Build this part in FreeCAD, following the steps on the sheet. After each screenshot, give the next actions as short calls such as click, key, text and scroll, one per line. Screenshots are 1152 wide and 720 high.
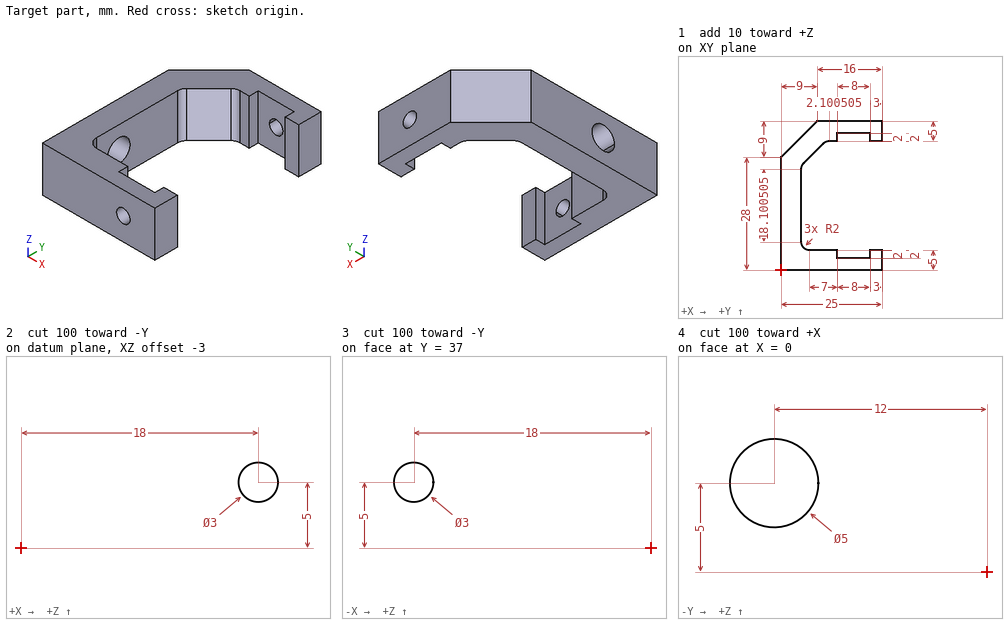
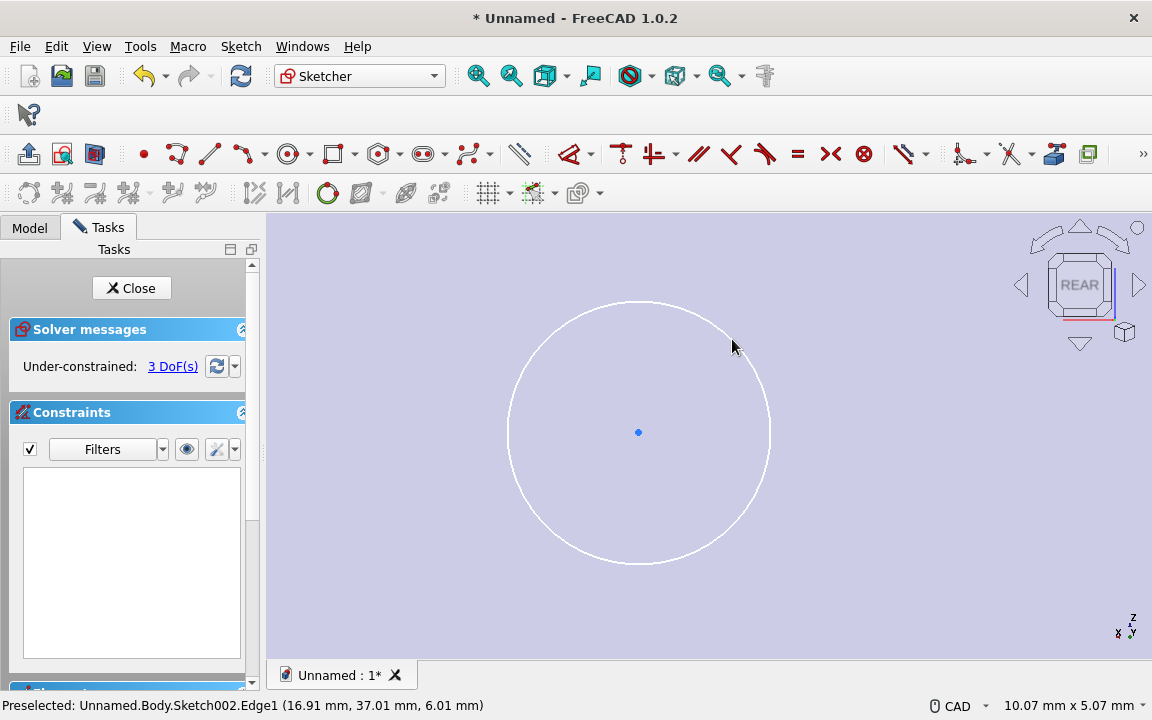
click(568, 154)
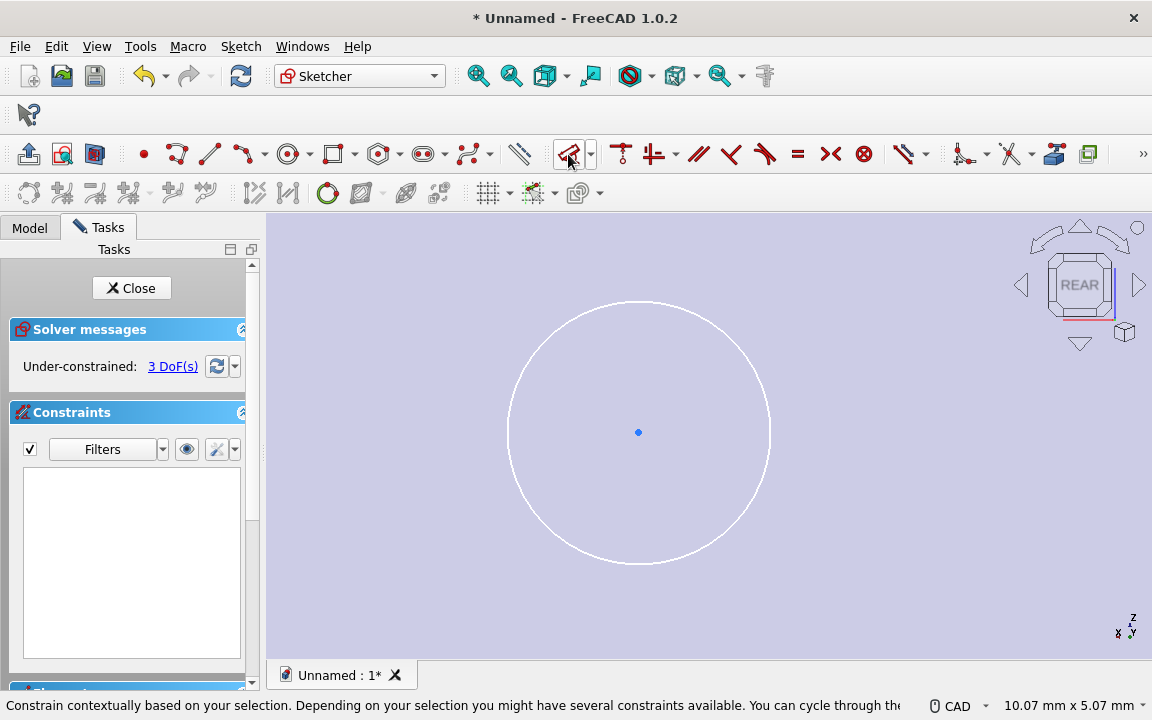
click(732, 340)
click(755, 317)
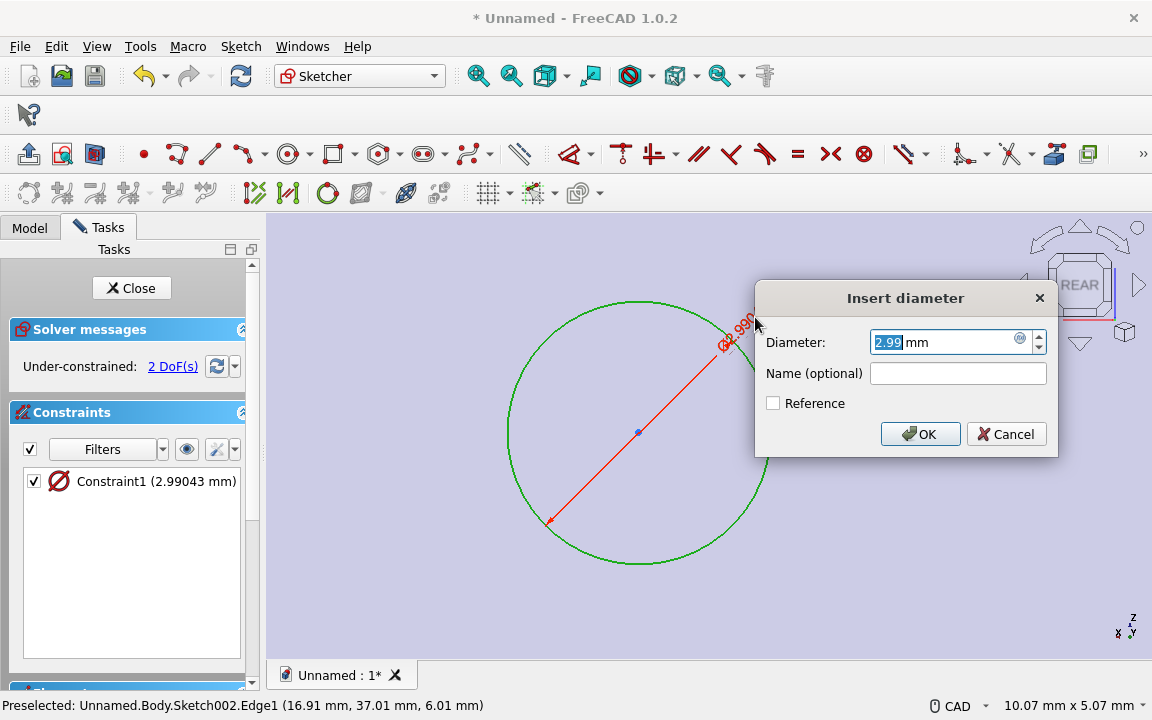
text(3)
key(Return)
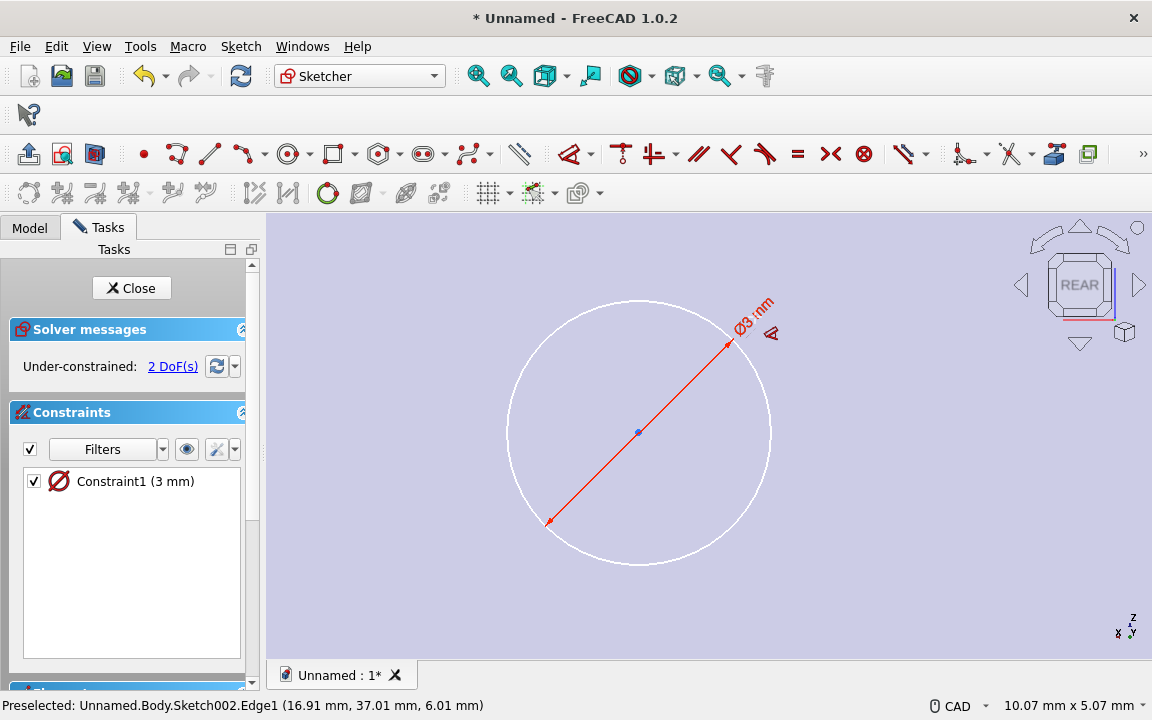
click(639, 433)
click(605, 532)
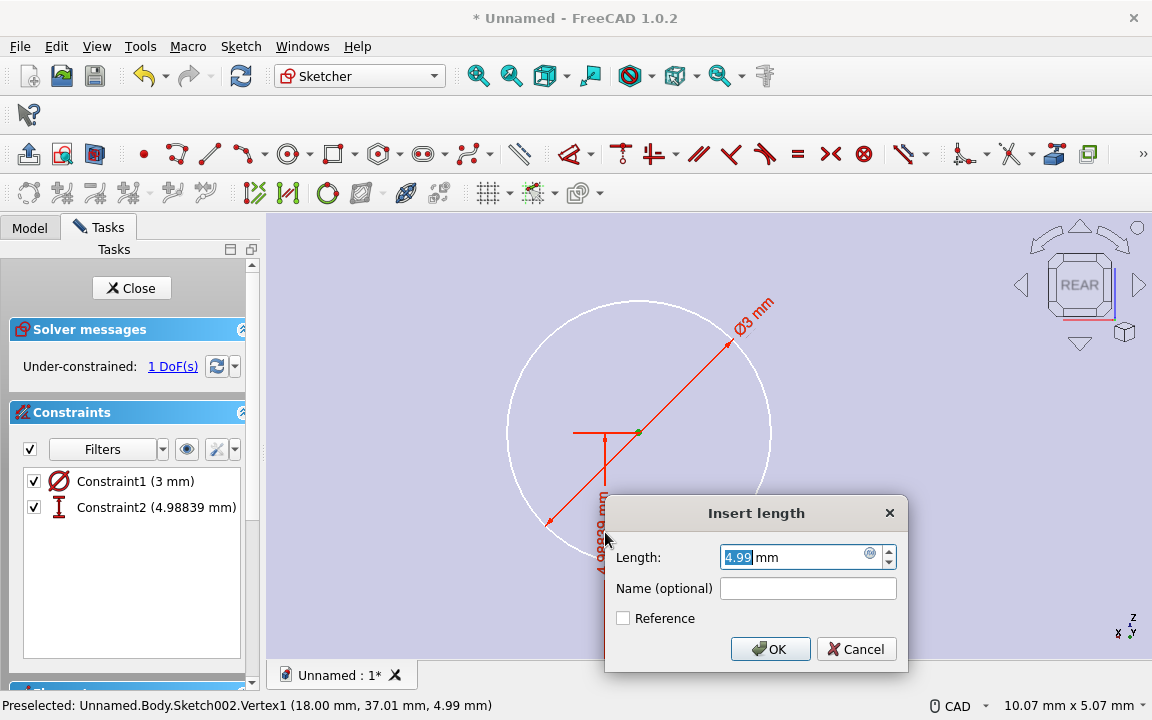
text(5)
key(Return)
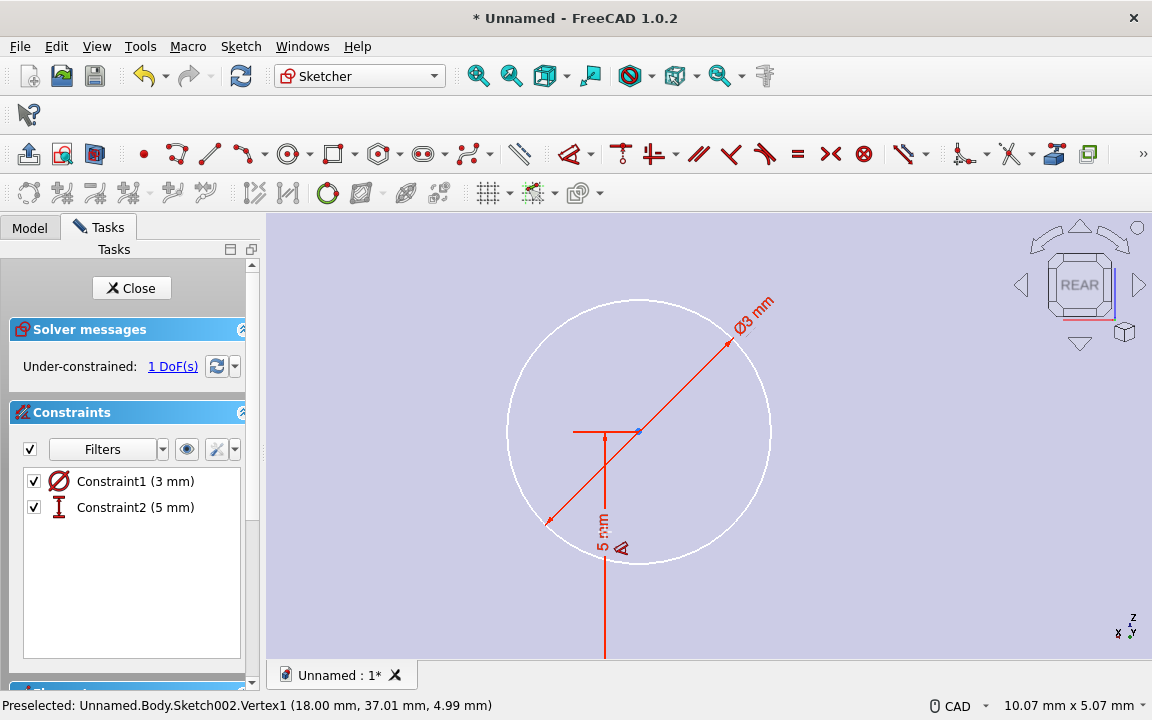
click(639, 432)
click(813, 398)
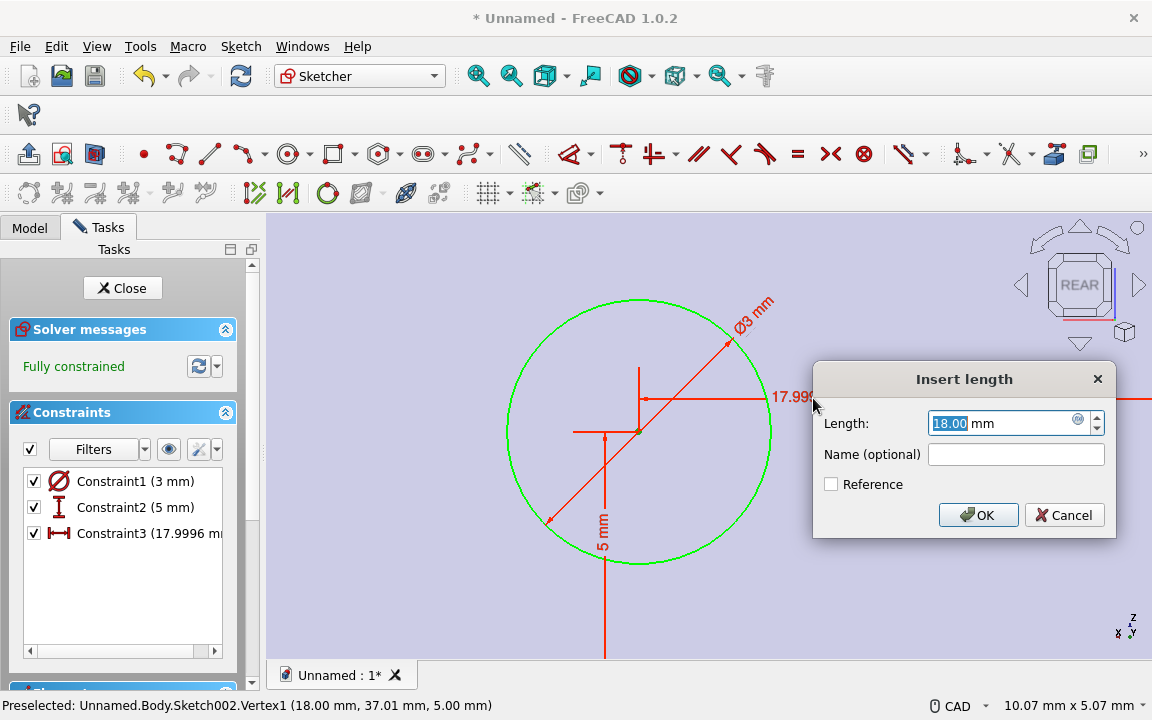
text(18)
key(Return)
key(Escape)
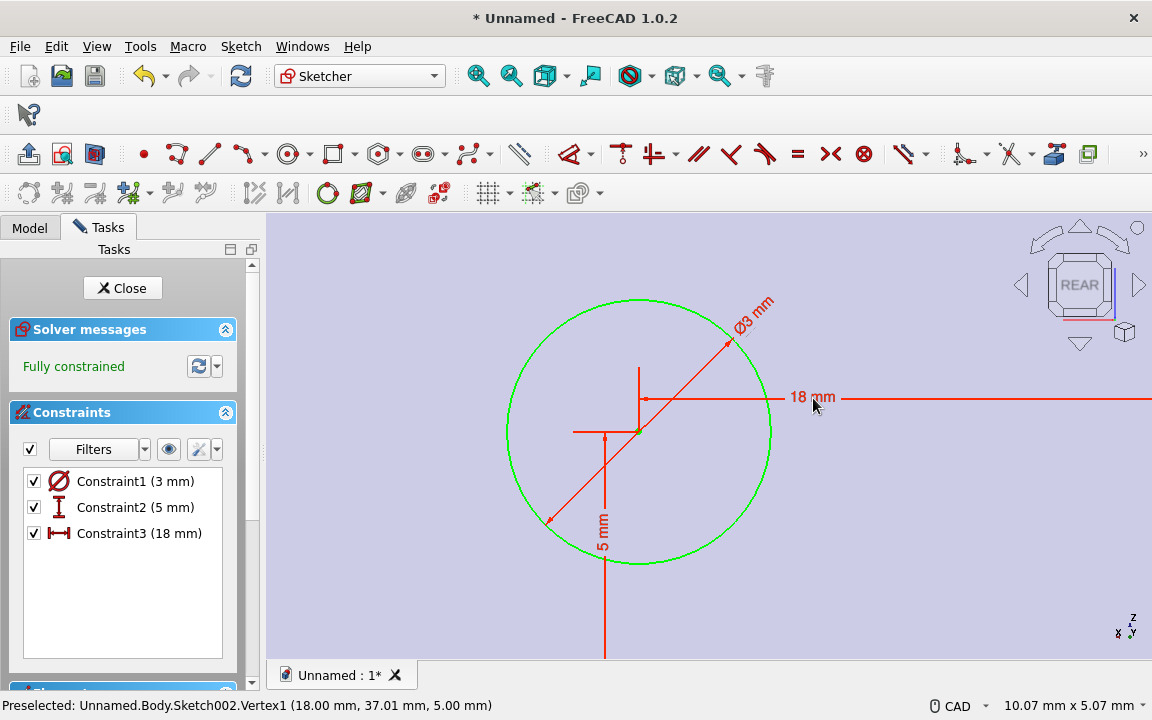
click(123, 288)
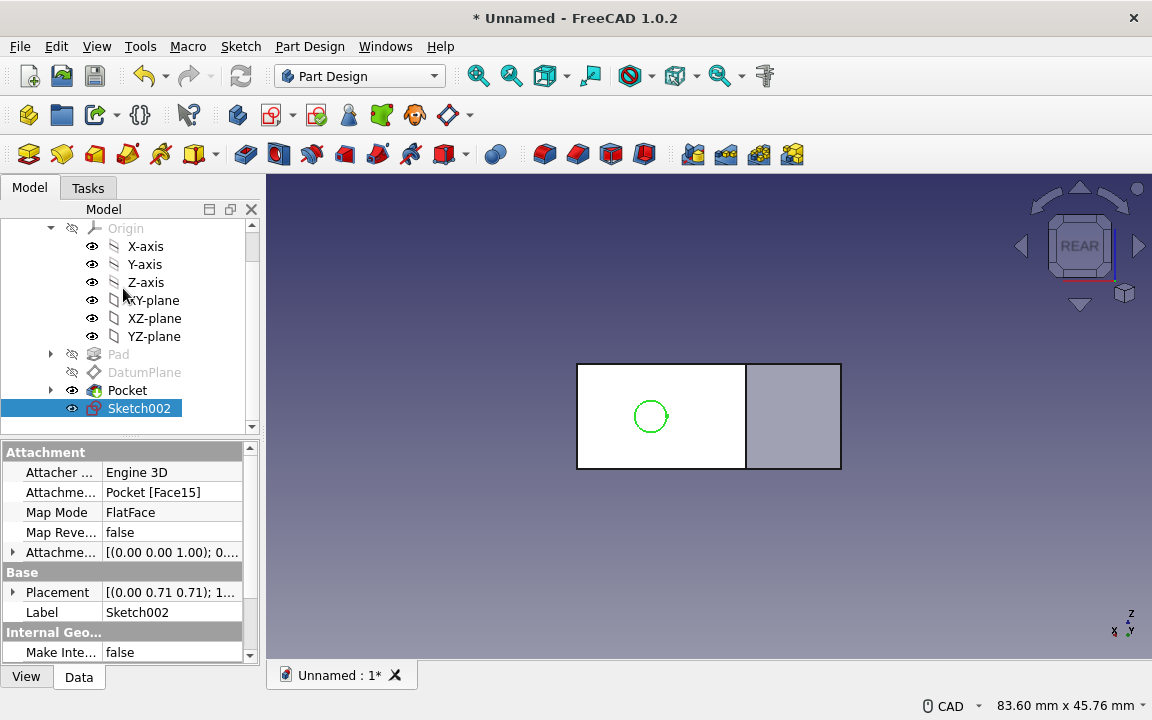
click(246, 154)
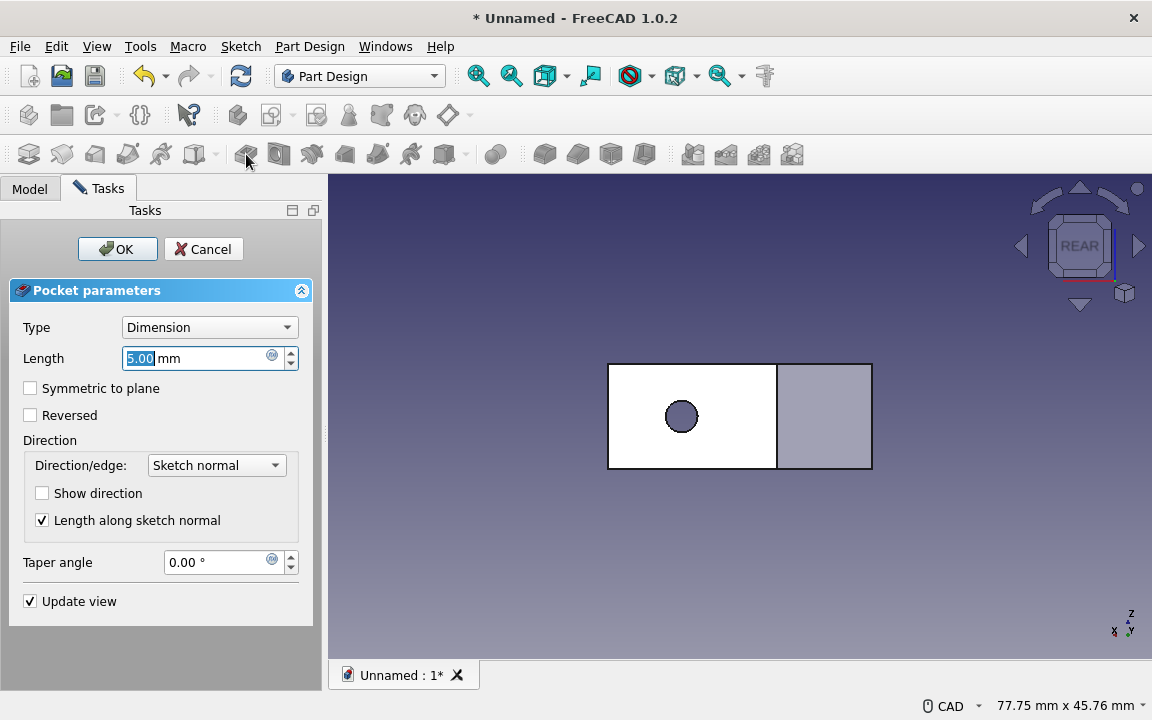
text(100)
key(Tab)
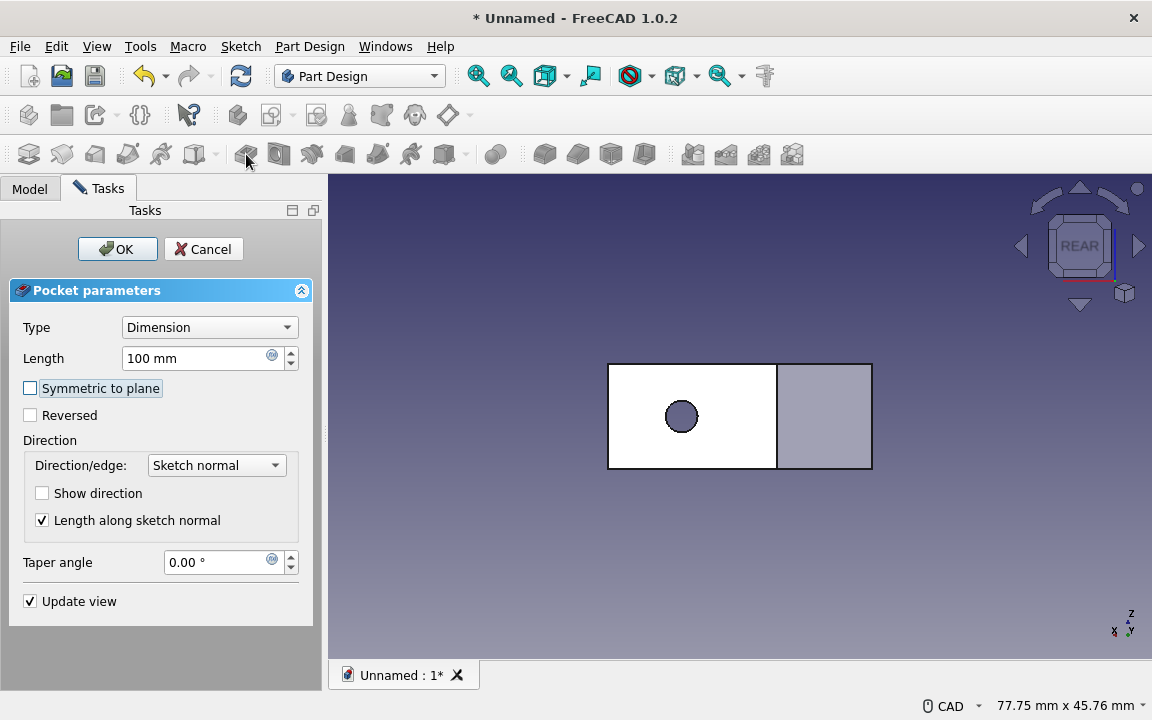
click(118, 249)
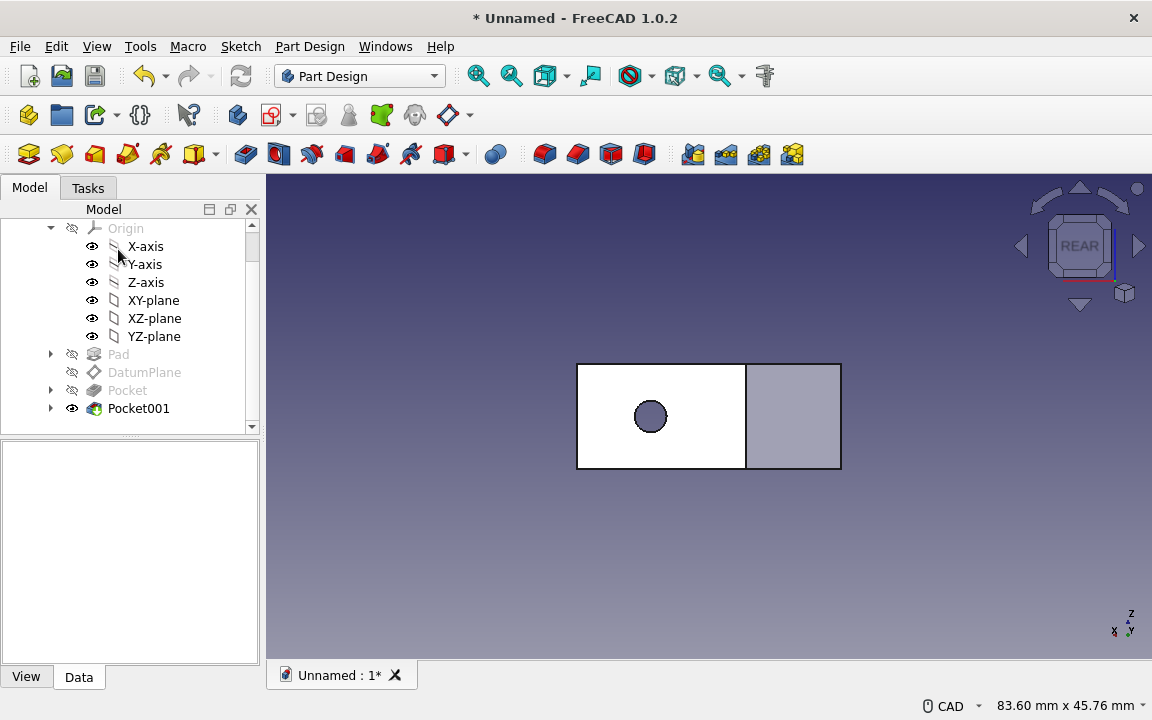
click(479, 76)